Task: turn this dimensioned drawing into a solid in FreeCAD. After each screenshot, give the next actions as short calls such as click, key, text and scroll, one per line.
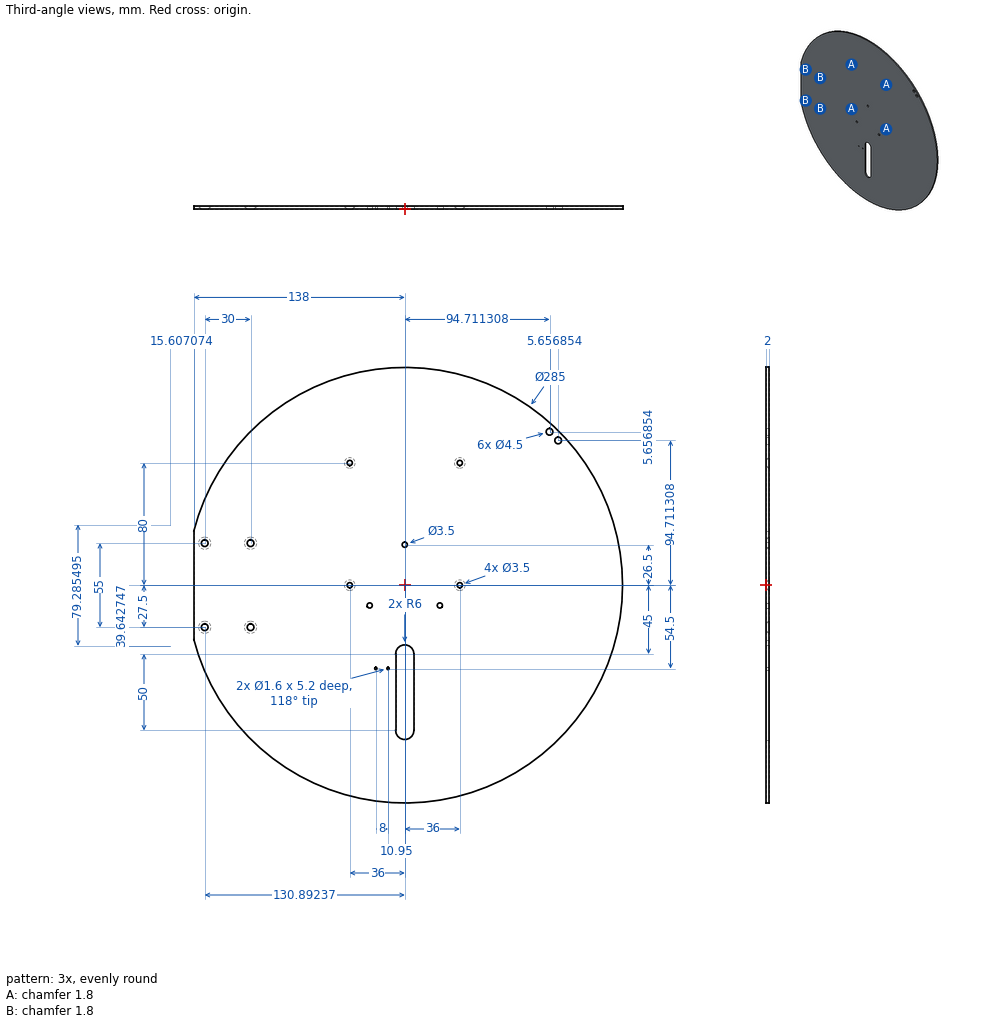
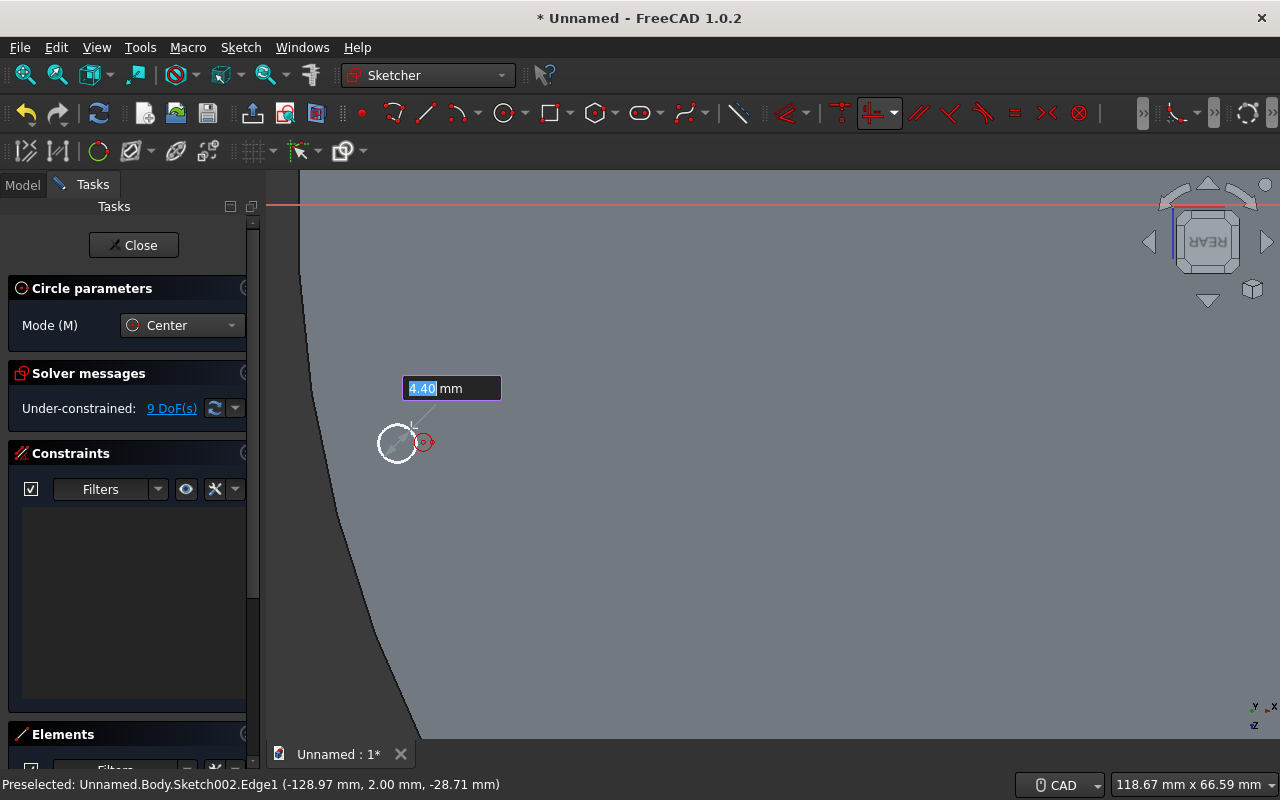
click(410, 427)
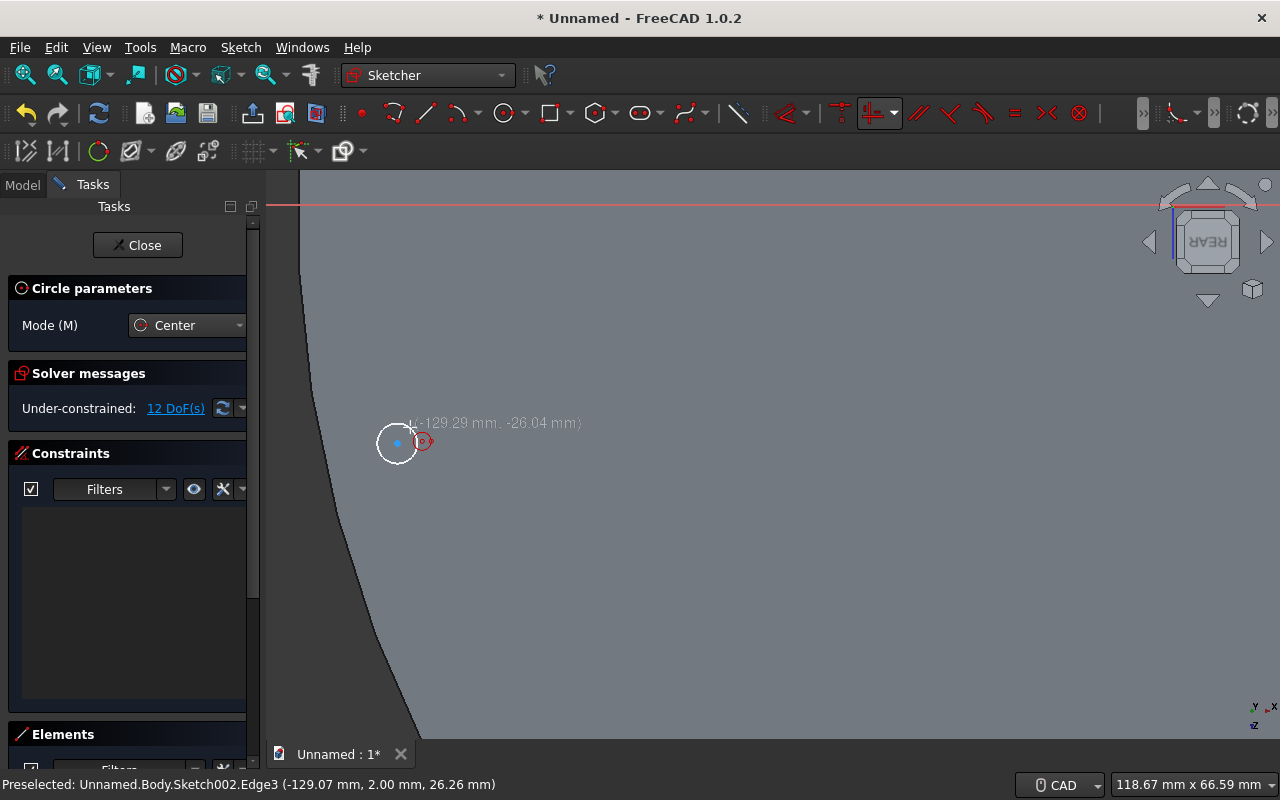
click(653, 440)
click(666, 427)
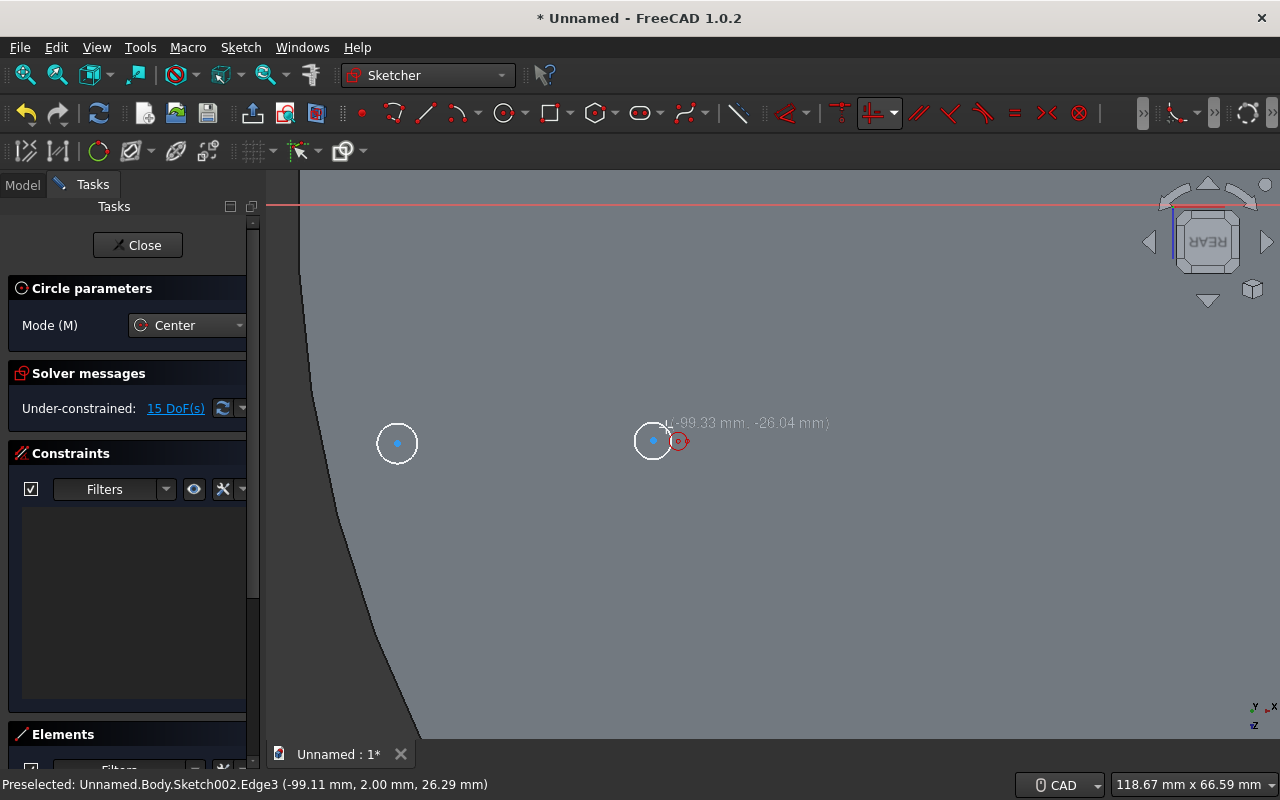
scroll(411, 428, down, 6)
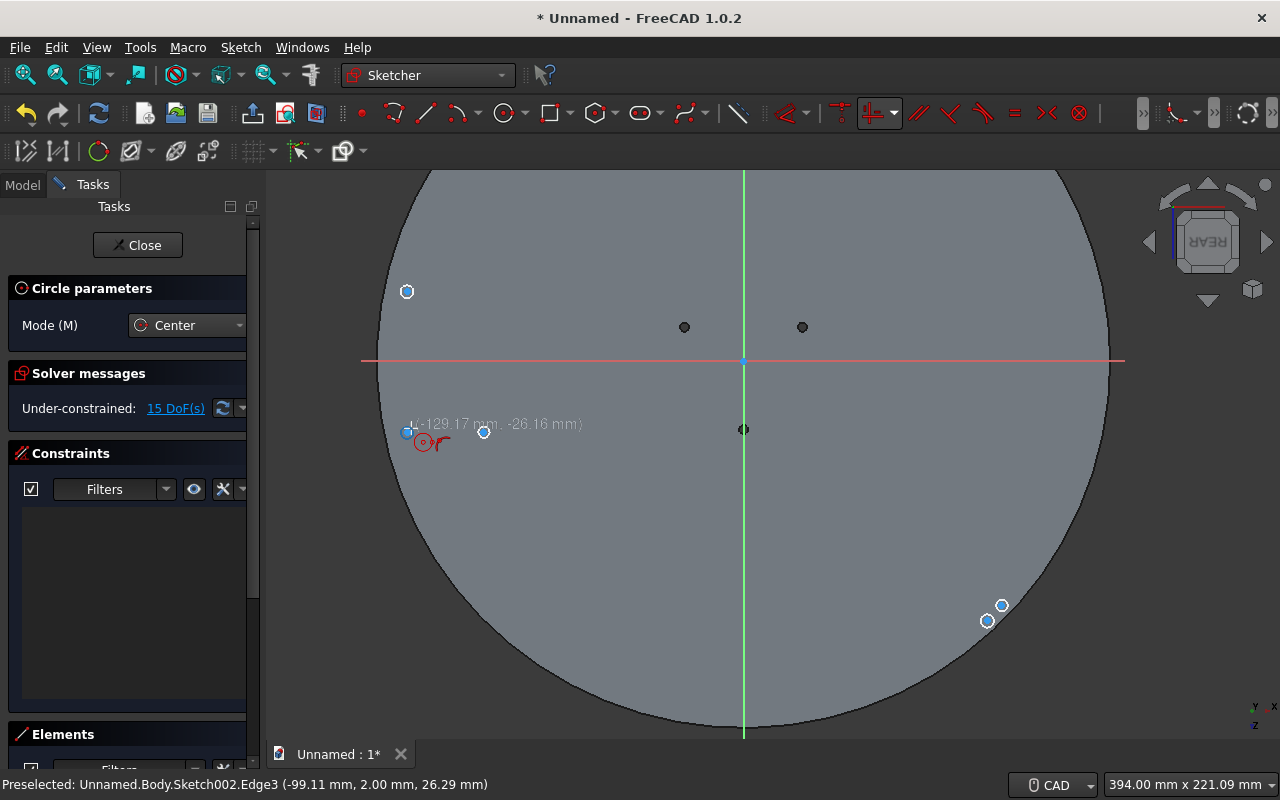
scroll(484, 291, up, 7)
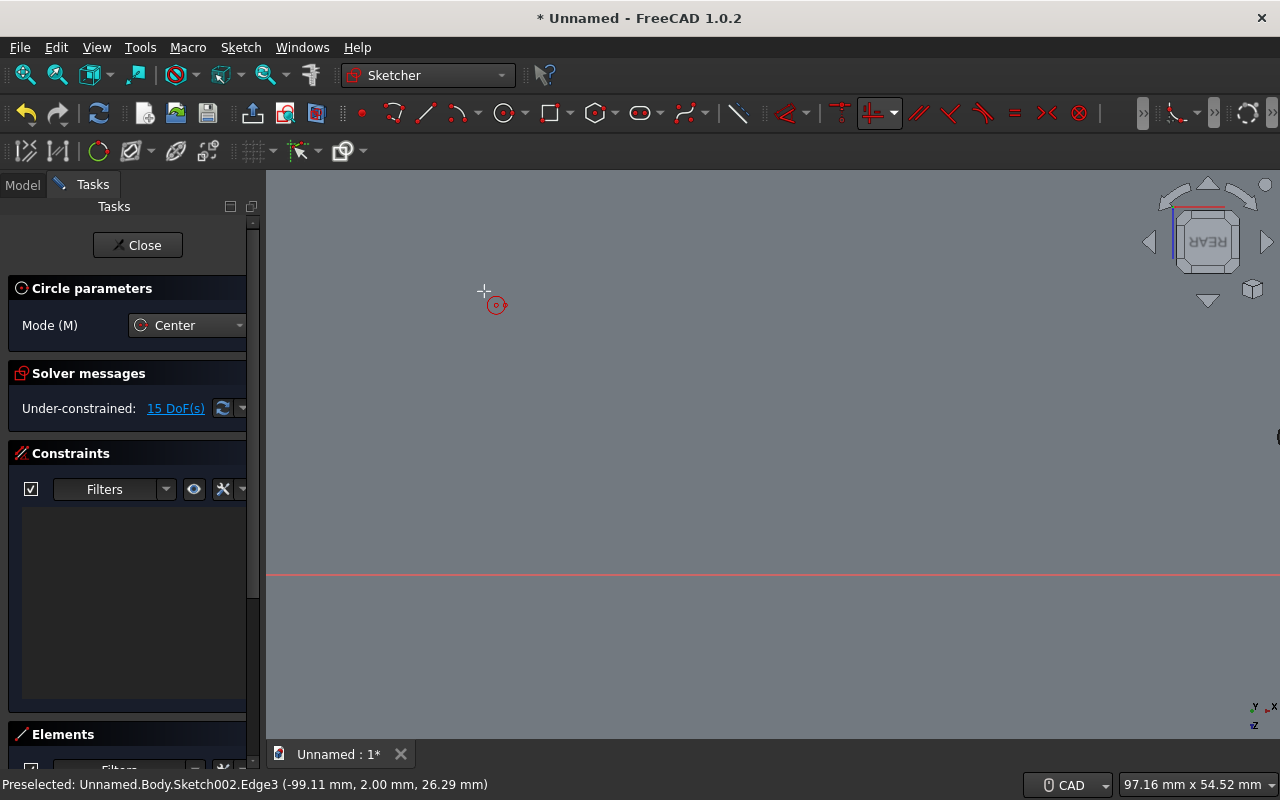
scroll(485, 290, down, 7)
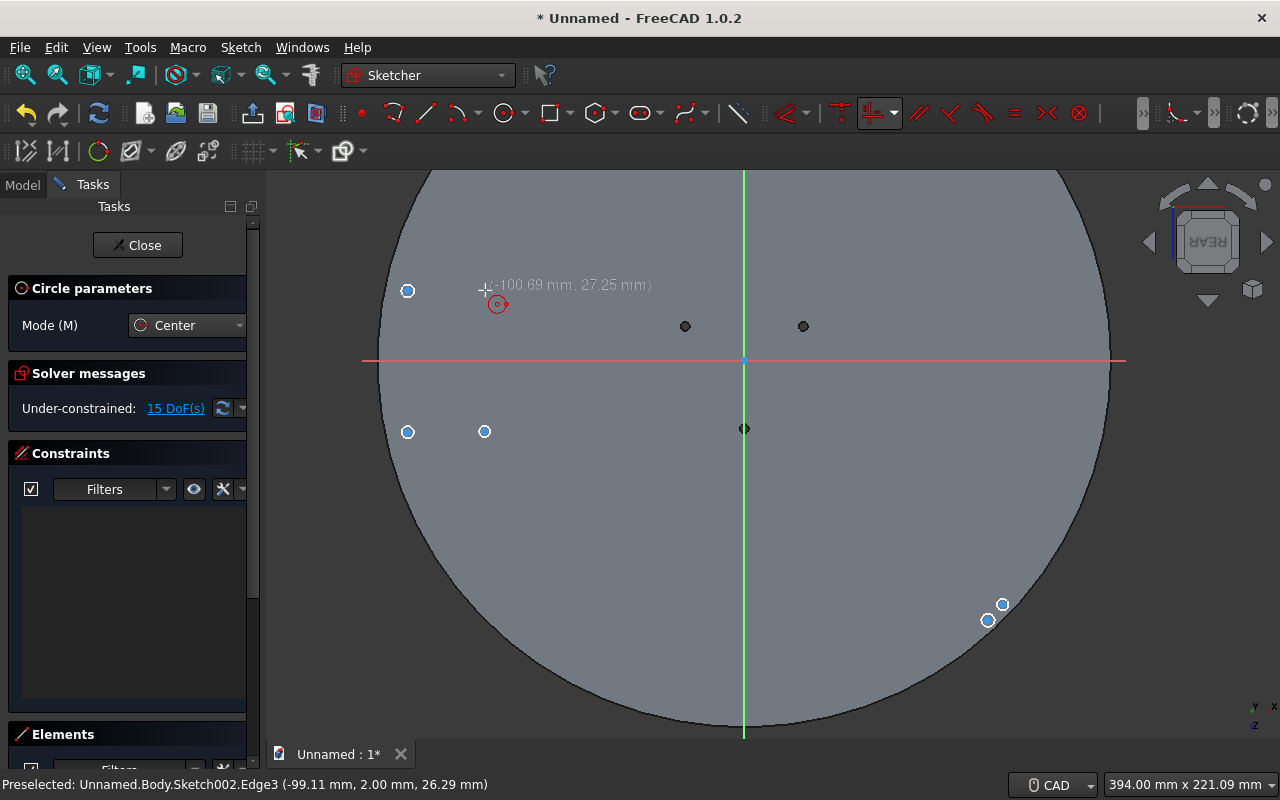
click(485, 290)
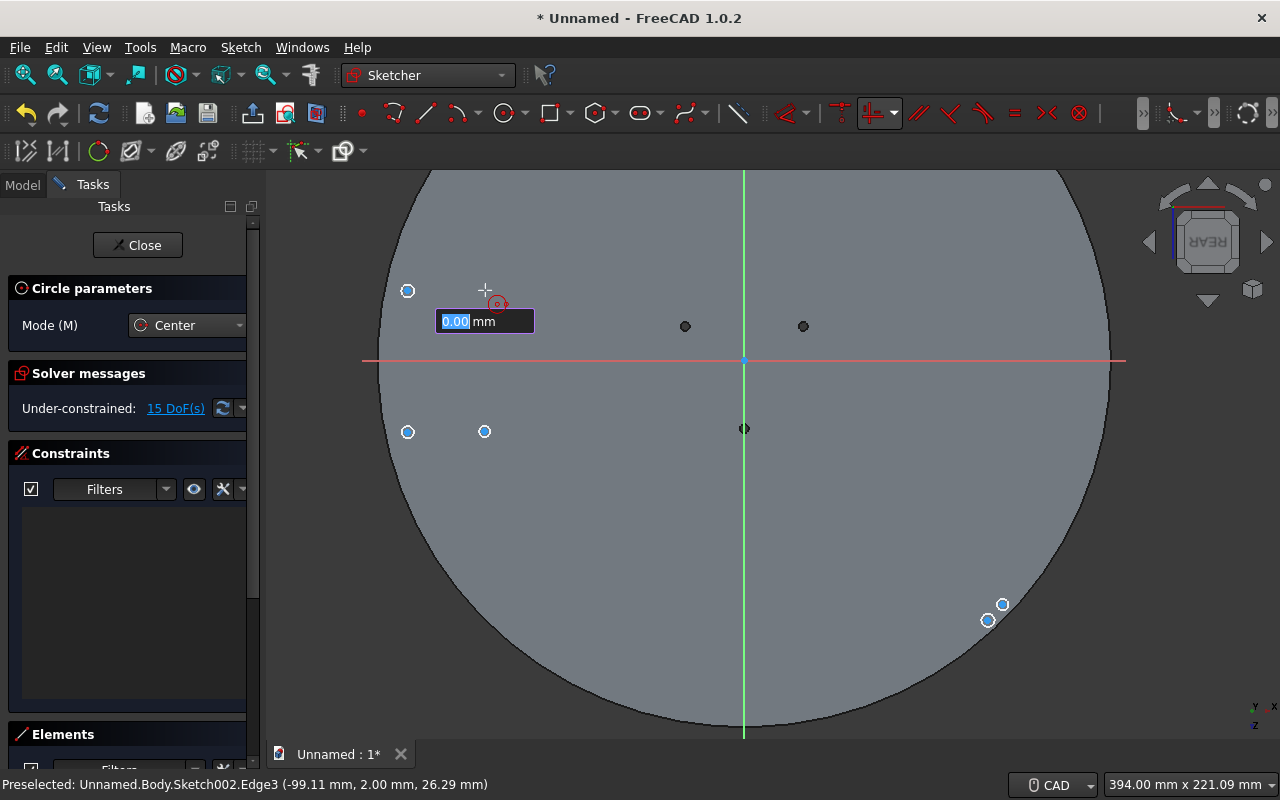
scroll(489, 286, up, 6)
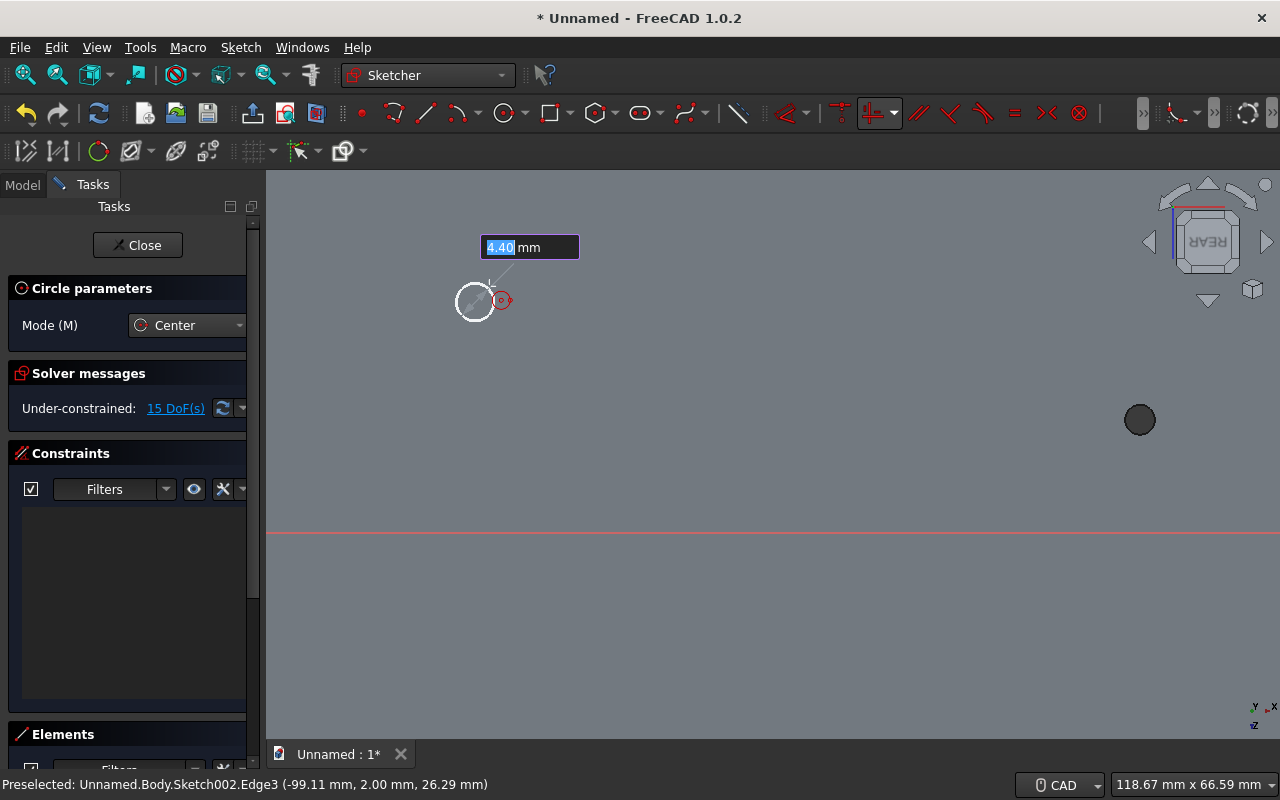
click(488, 284)
key(Escape)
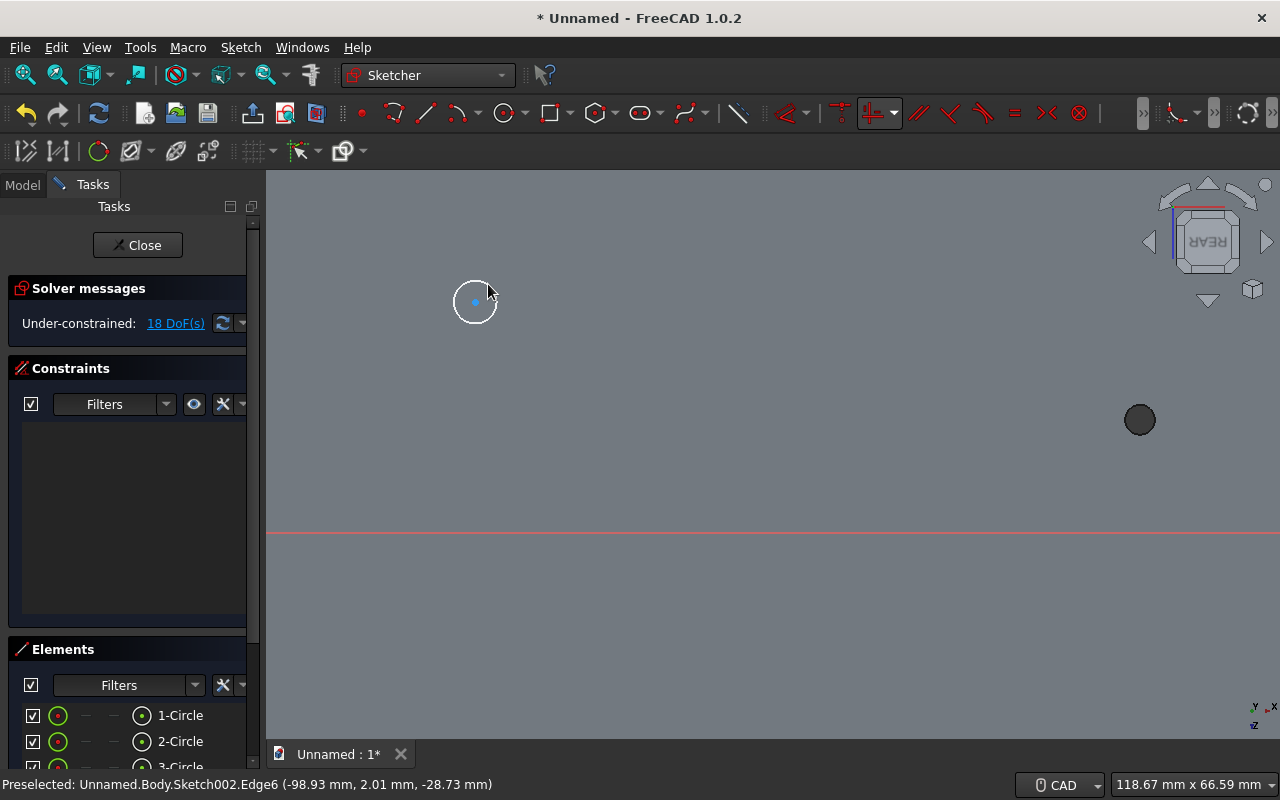
scroll(488, 286, down, 6)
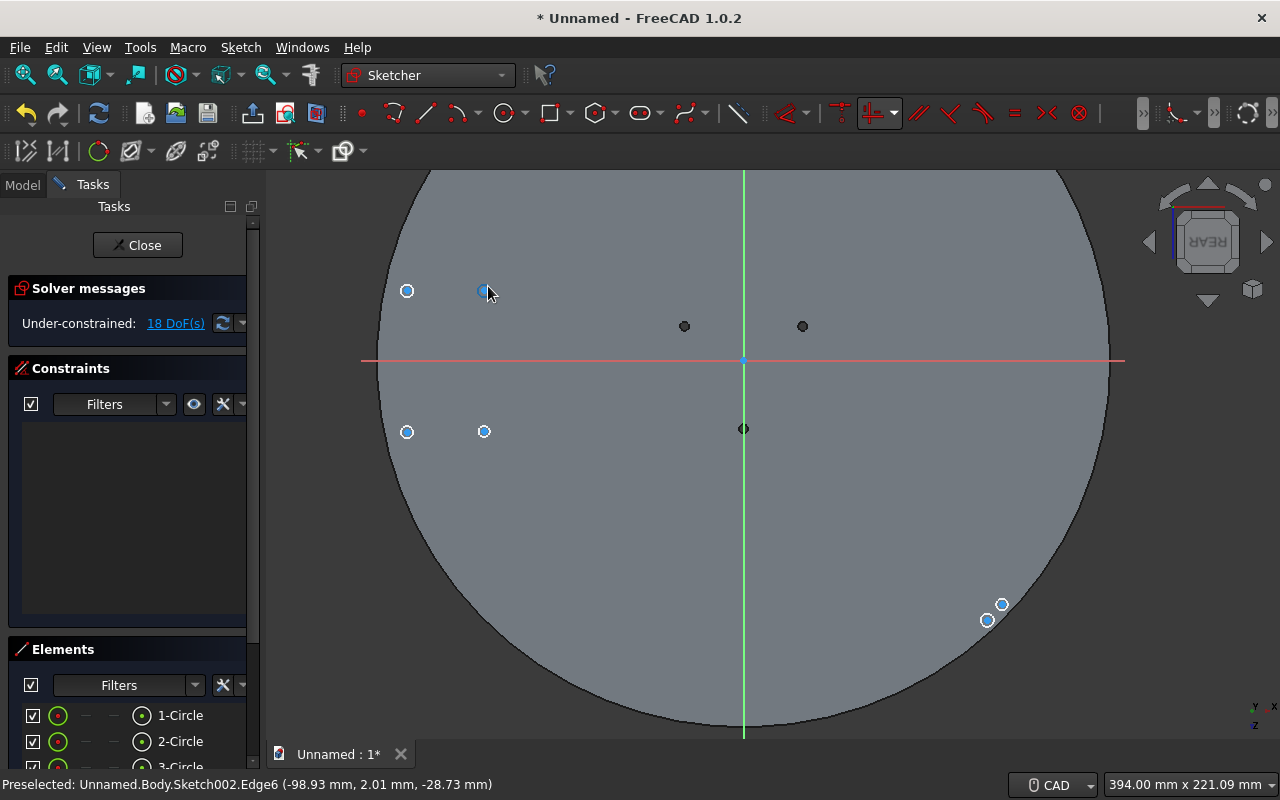
scroll(992, 616, up, 4)